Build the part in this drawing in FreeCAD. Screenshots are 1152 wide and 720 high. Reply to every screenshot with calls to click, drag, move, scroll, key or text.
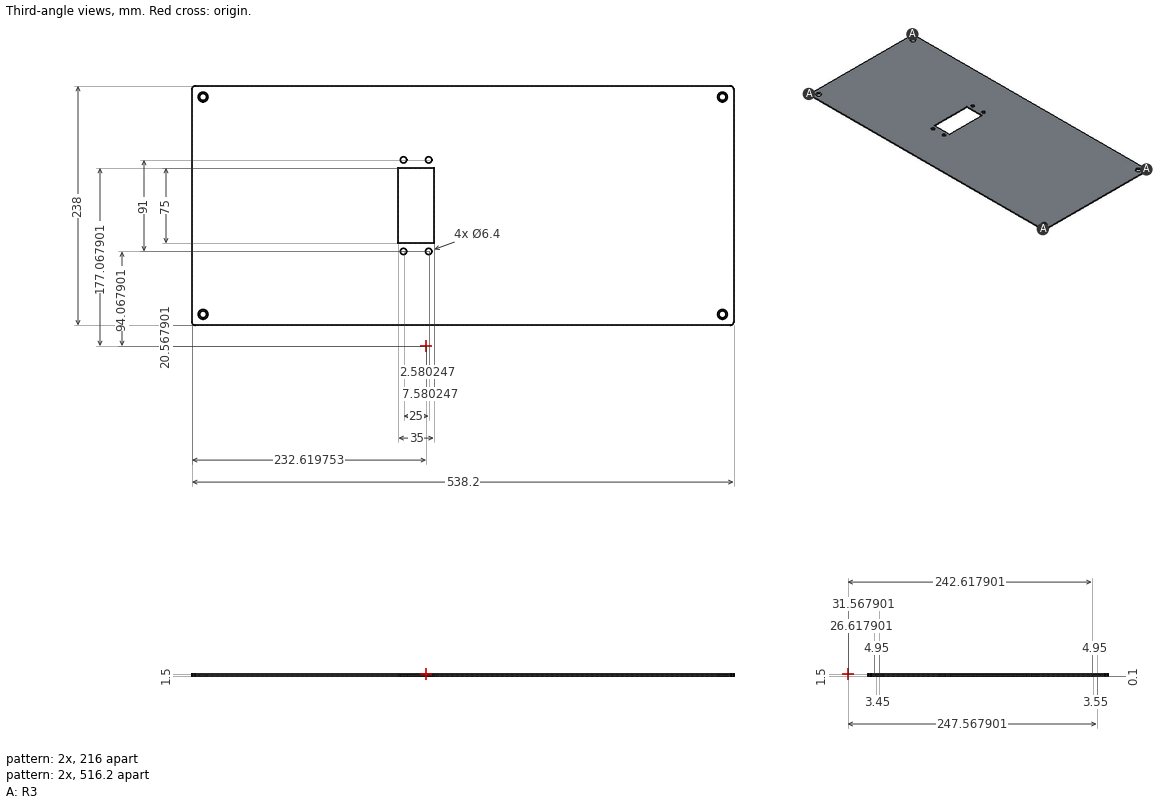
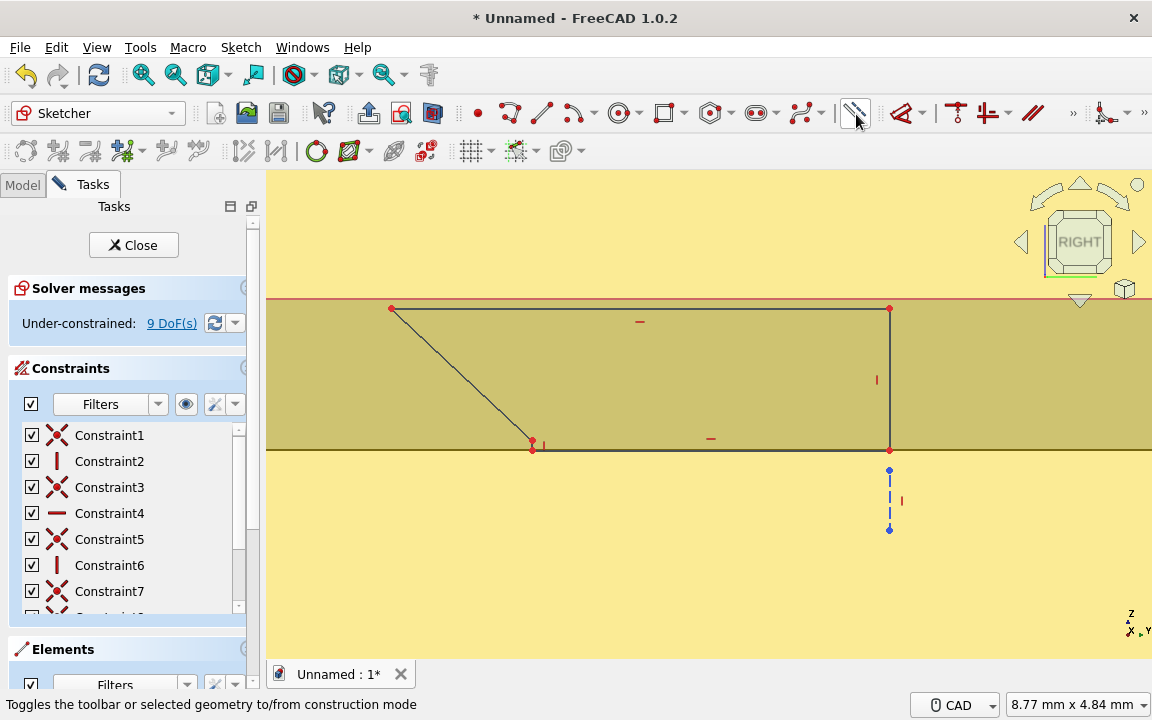
click(391, 309)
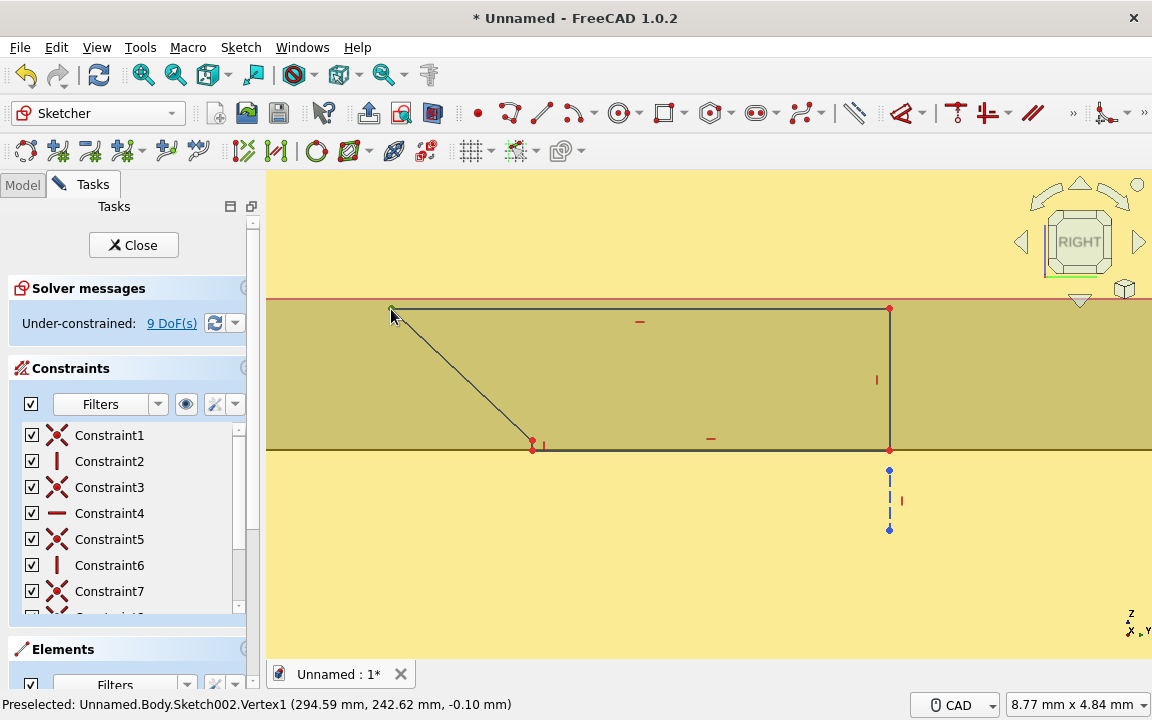
click(343, 299)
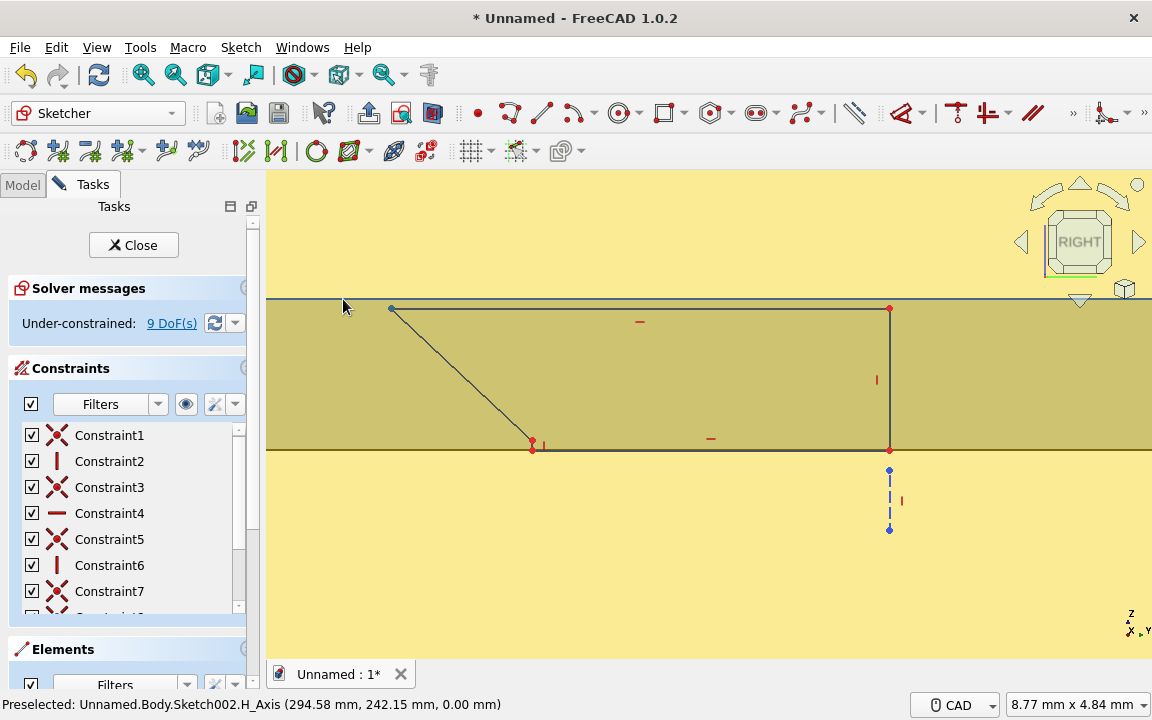
key(c)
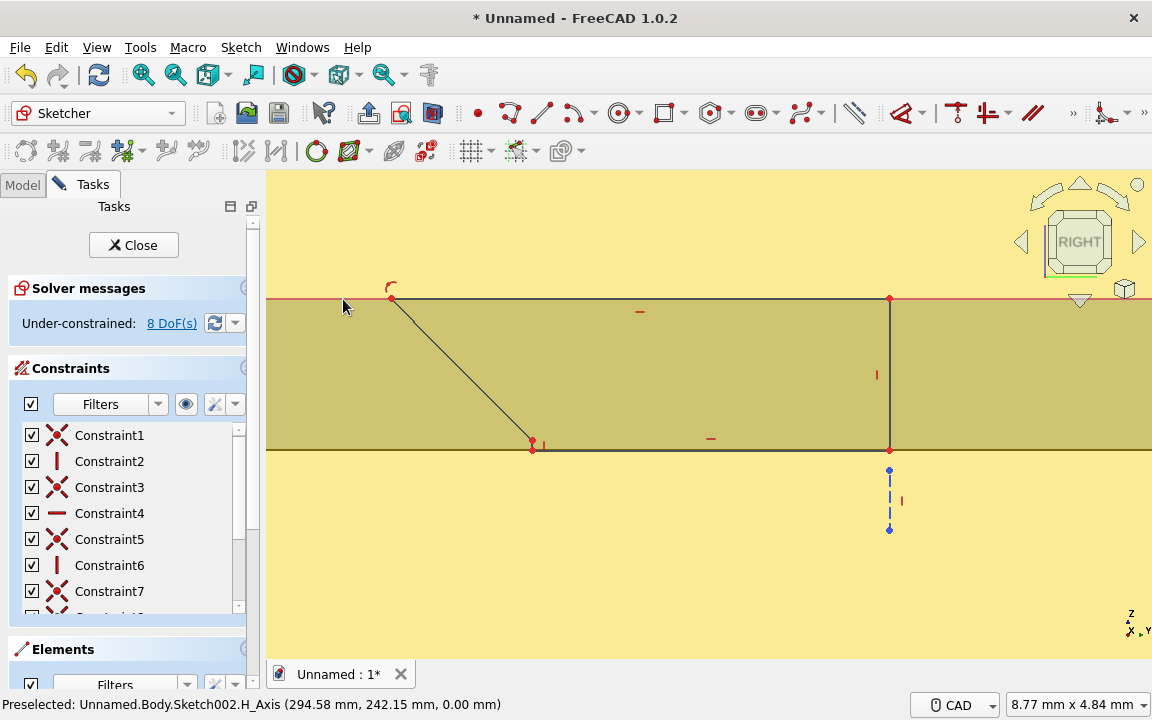
click(902, 114)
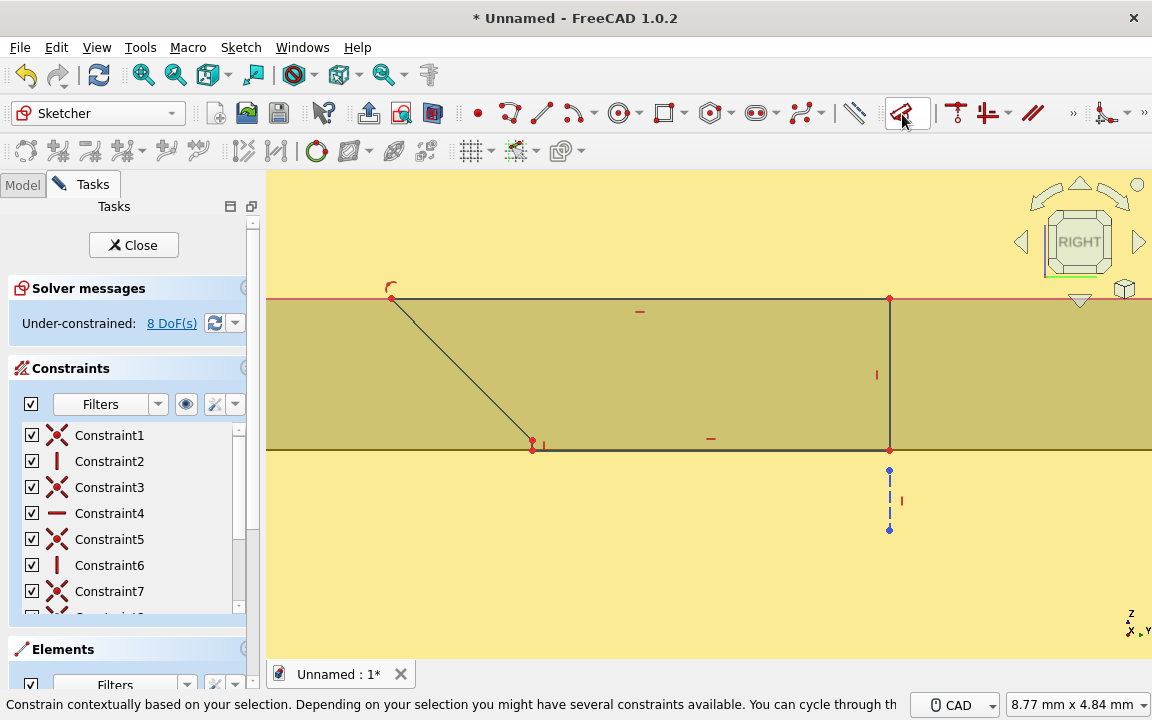
scroll(532, 446, up, 7)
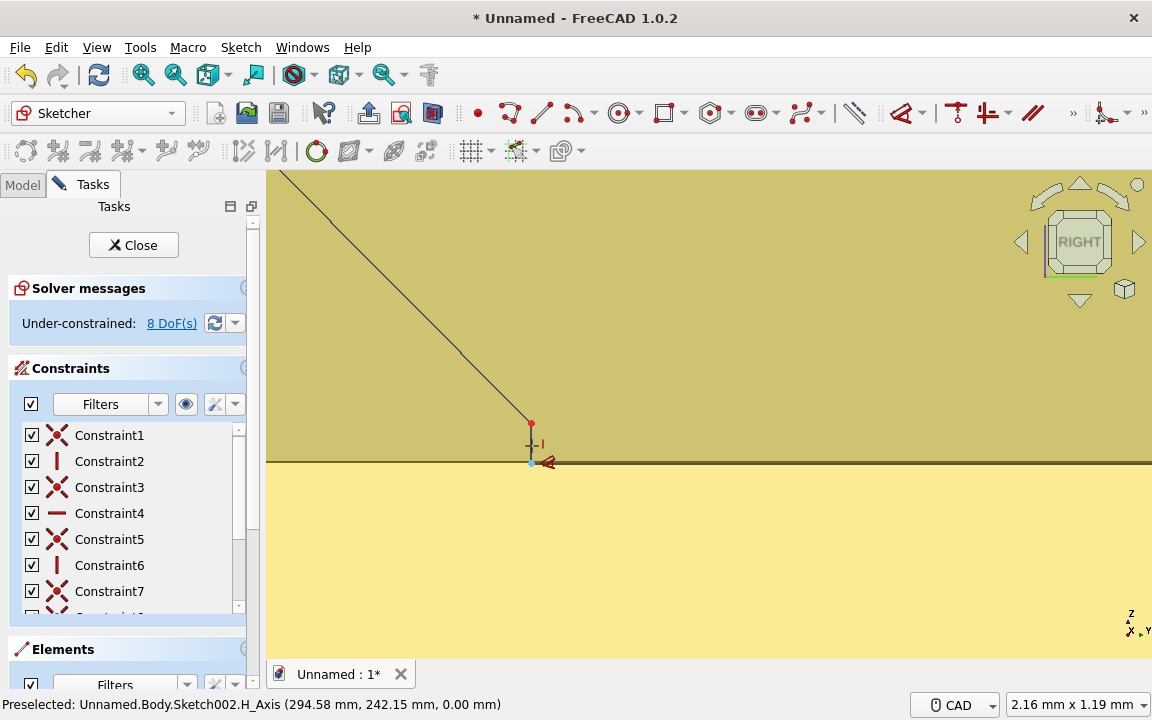
click(531, 444)
click(497, 444)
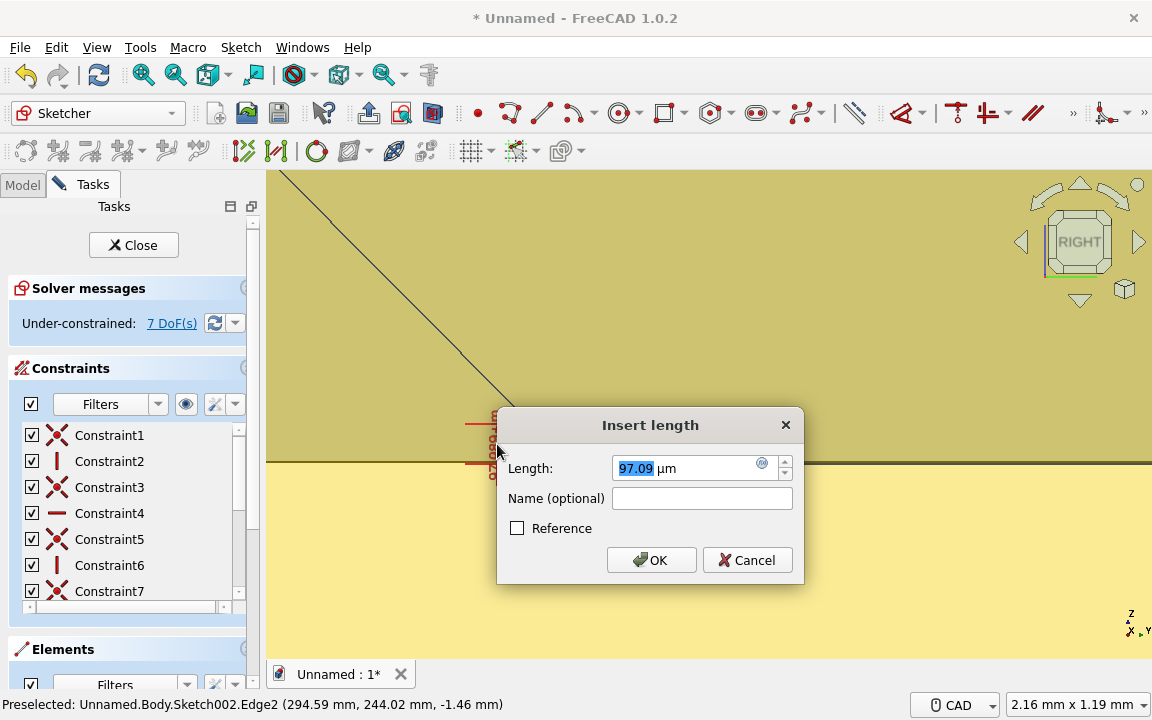
key(ctrl+a)
text(0.1 mm)
key(Return)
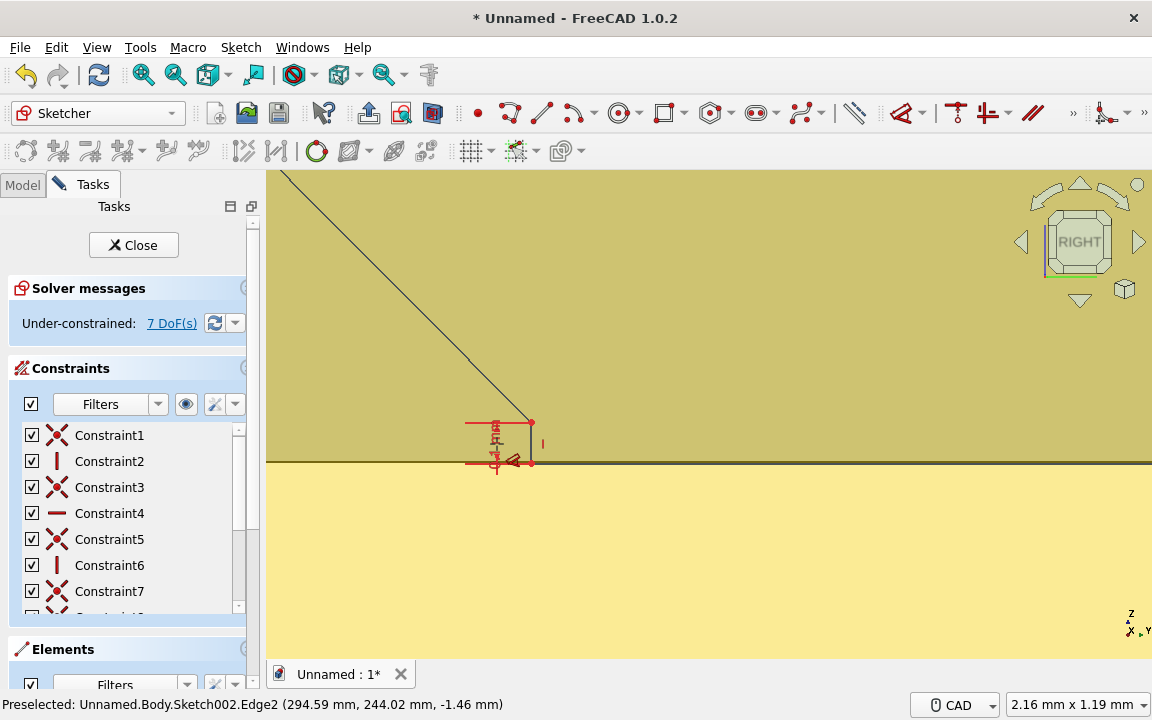
scroll(532, 446, down, 7)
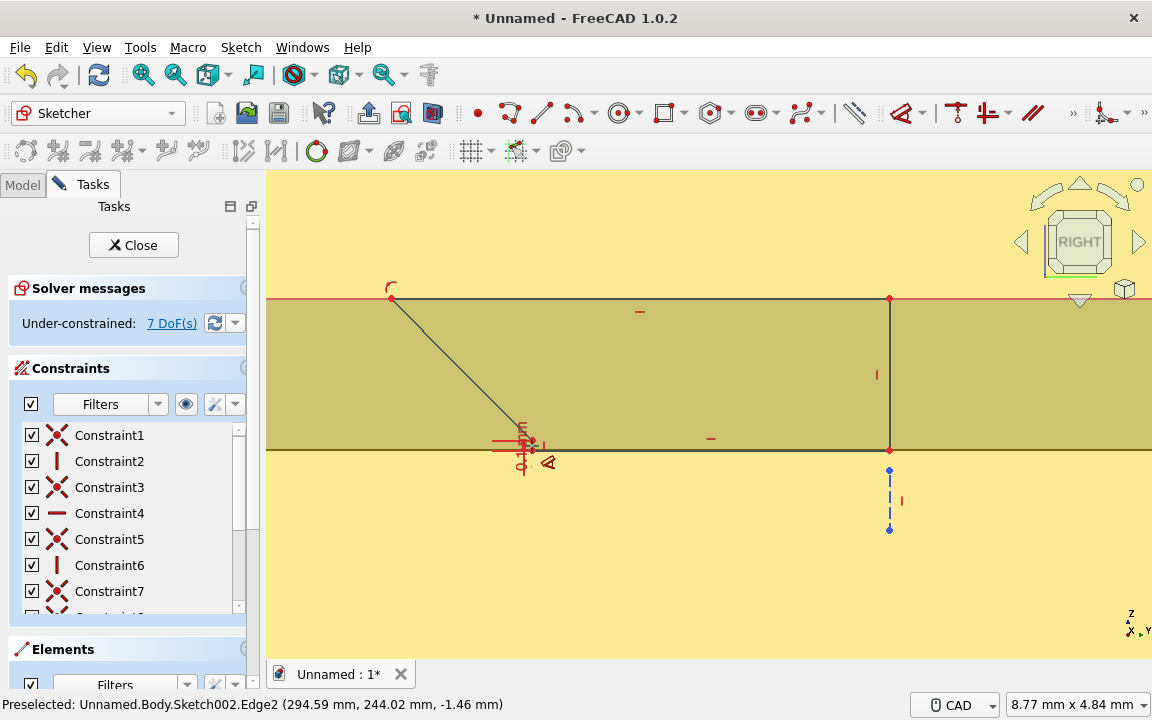
click(890, 405)
click(924, 375)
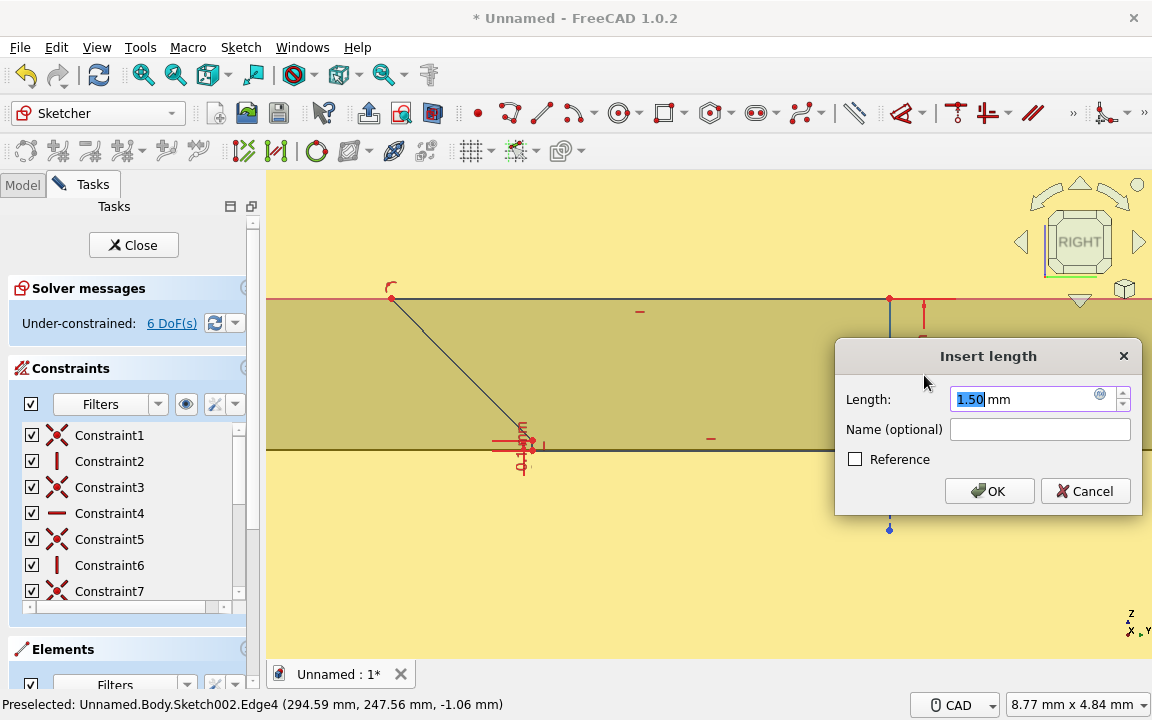
text(1.5)
key(Return)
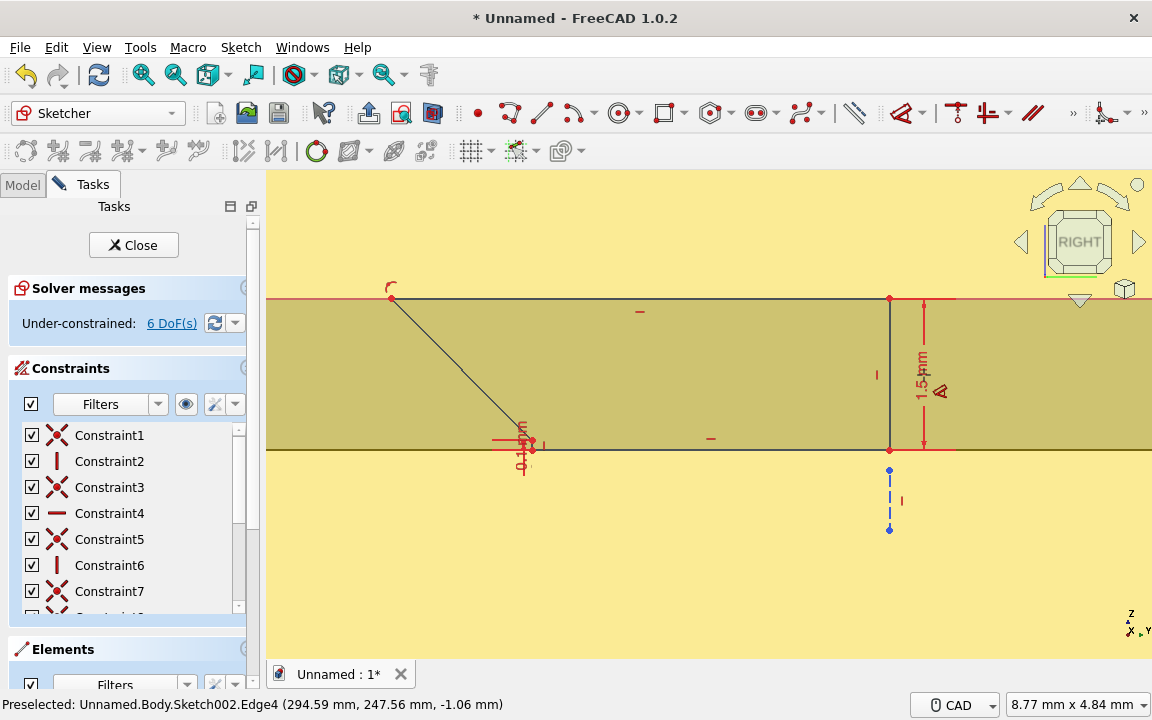
click(639, 450)
click(711, 484)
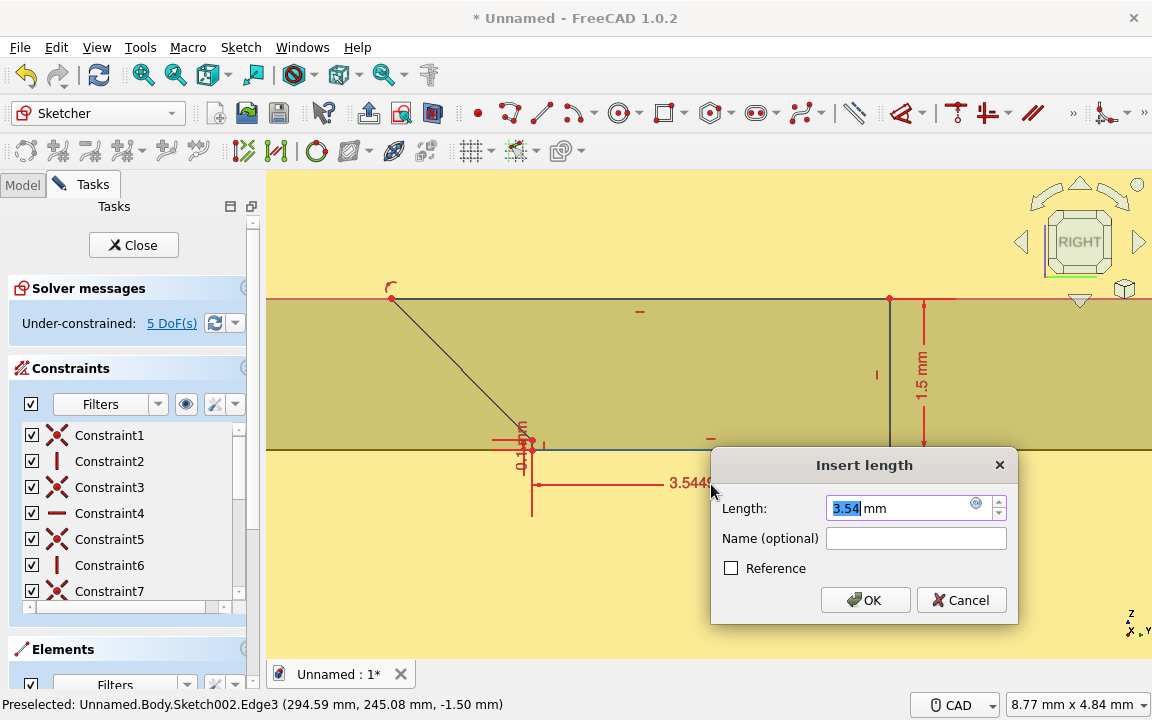
text(3.55)
key(Return)